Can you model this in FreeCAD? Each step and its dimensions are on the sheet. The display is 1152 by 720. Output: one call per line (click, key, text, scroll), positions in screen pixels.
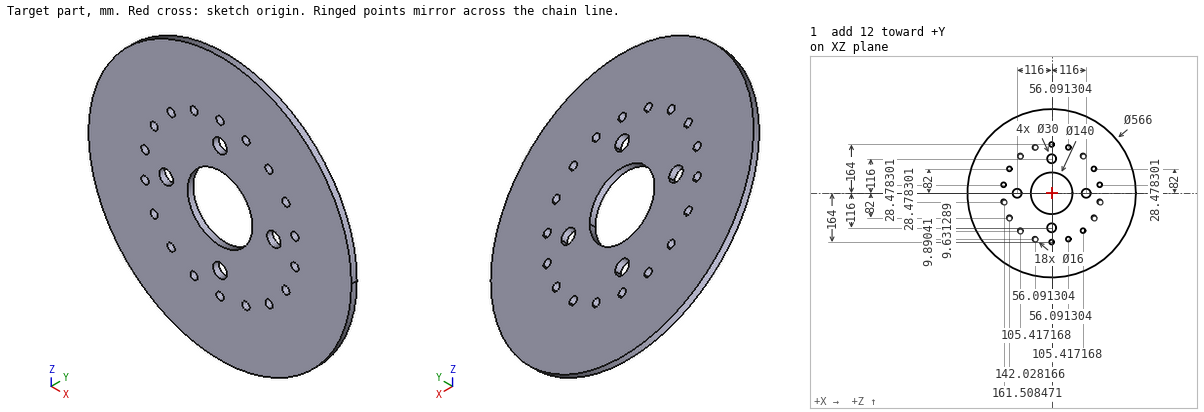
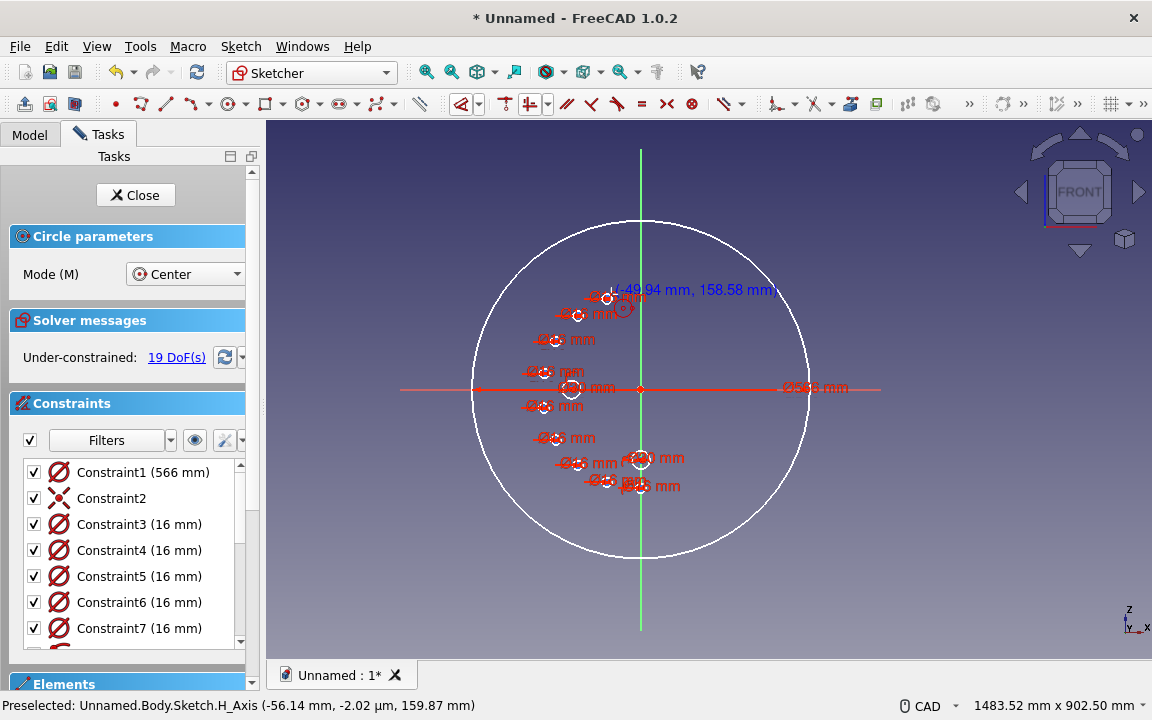
scroll(674, 482, up, 8)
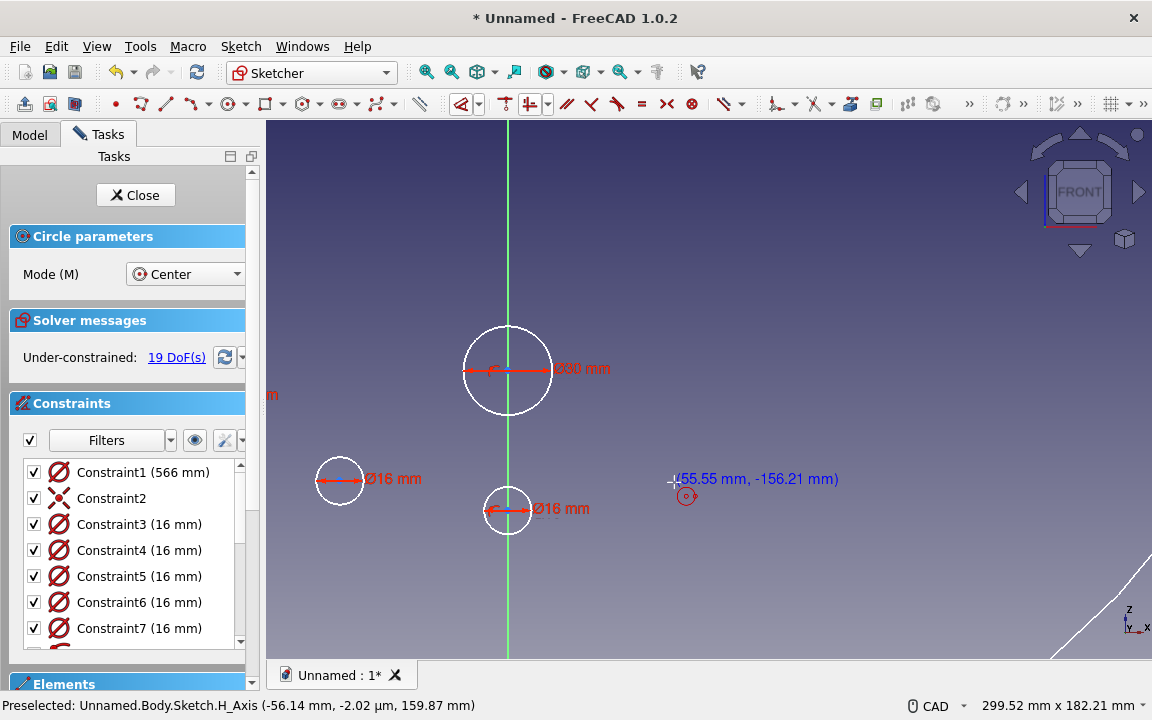
scroll(674, 482, down, 8)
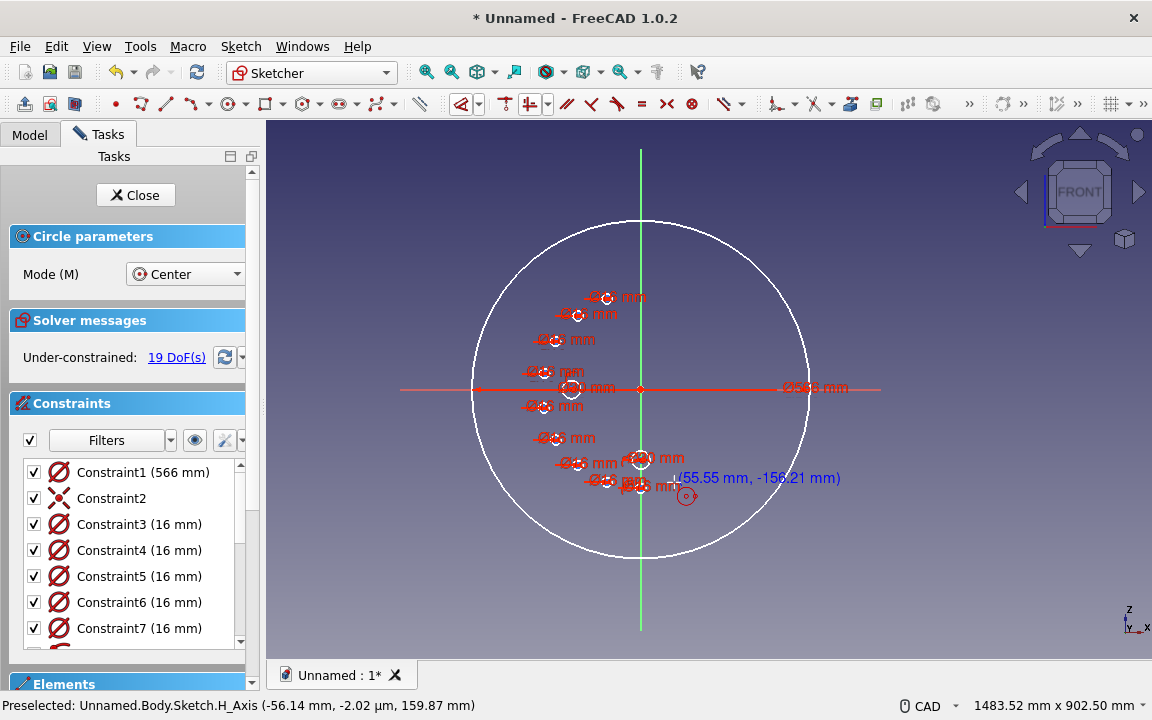
click(674, 482)
move(678, 478)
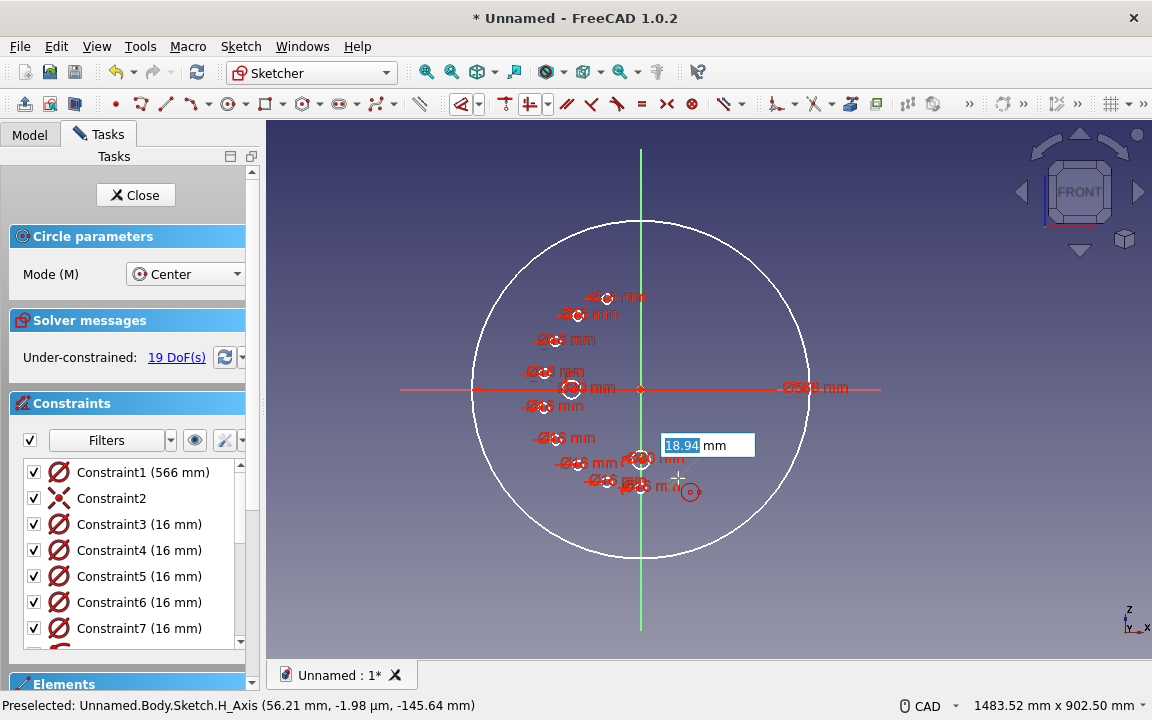
text(16)
key(Return)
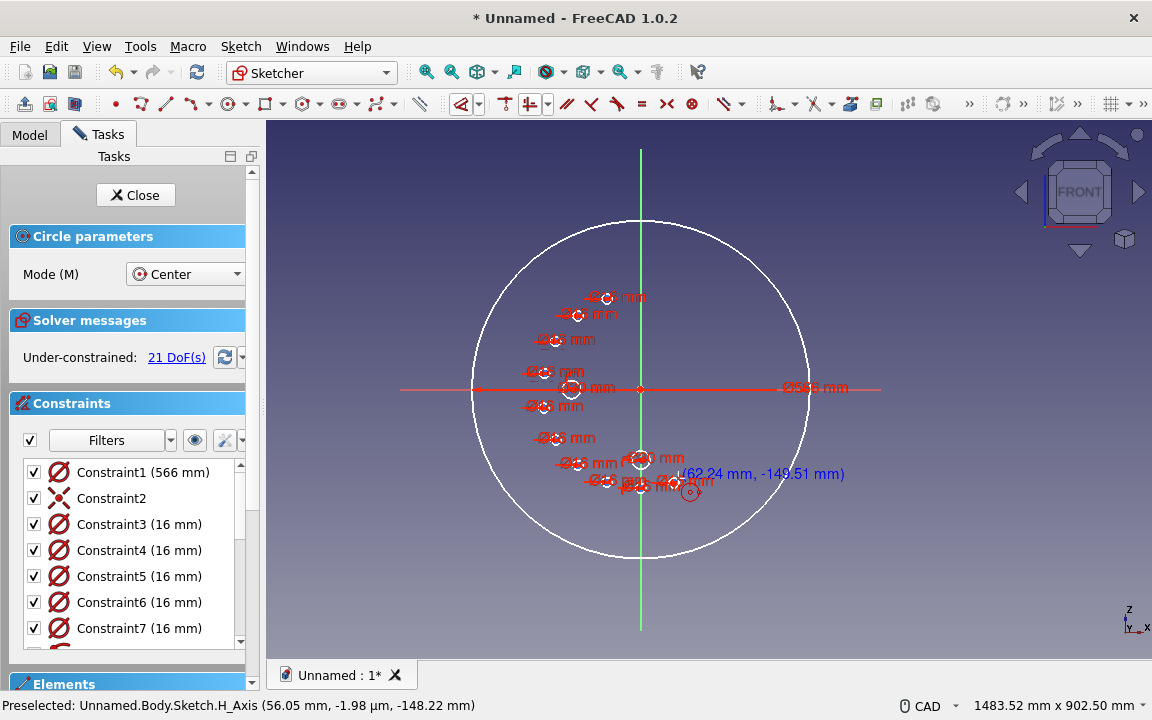
scroll(704, 465, up, 8)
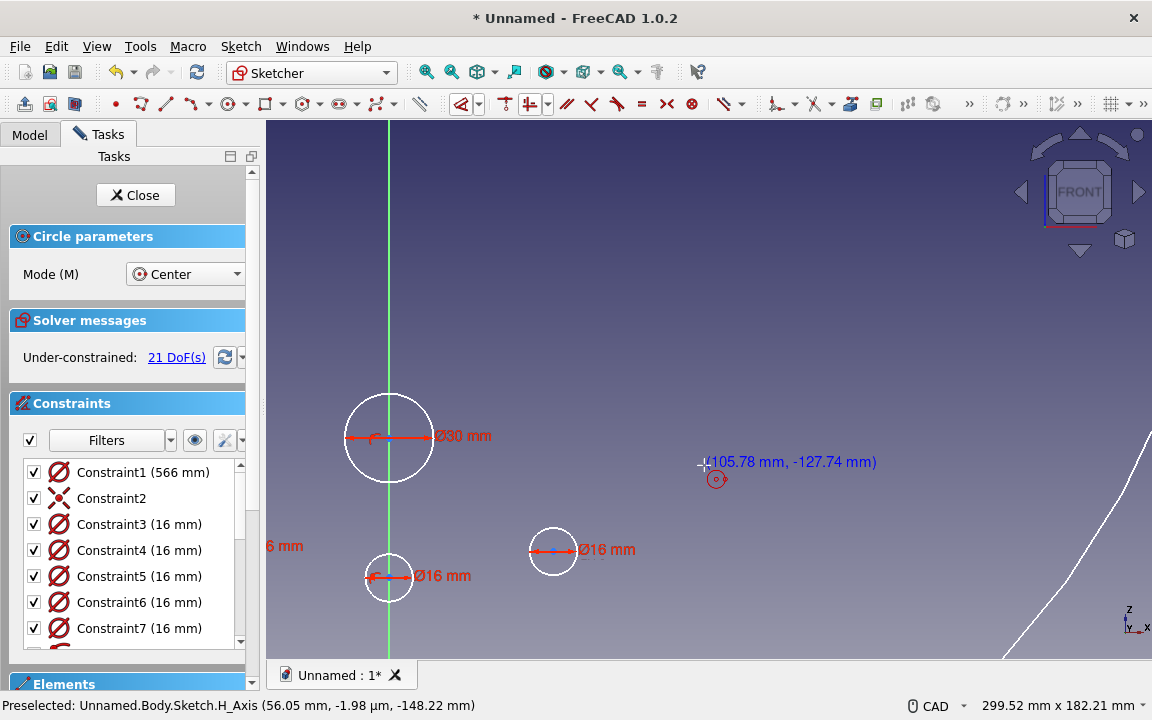
scroll(704, 465, down, 8)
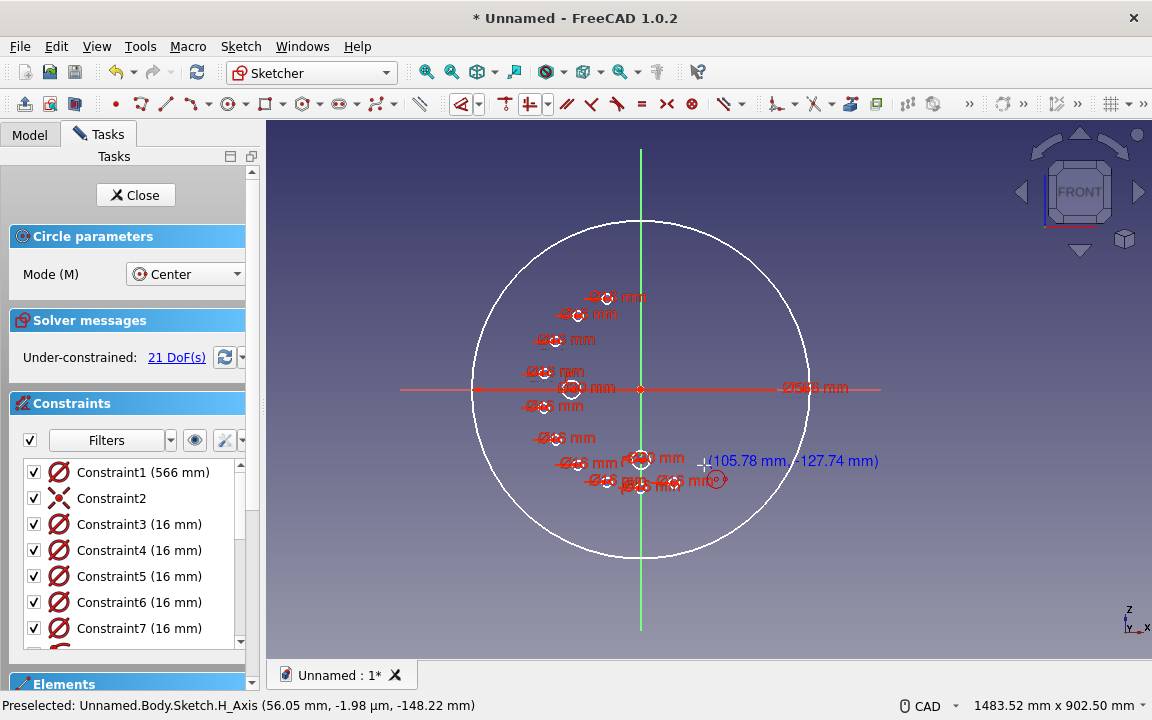
click(704, 465)
move(707, 461)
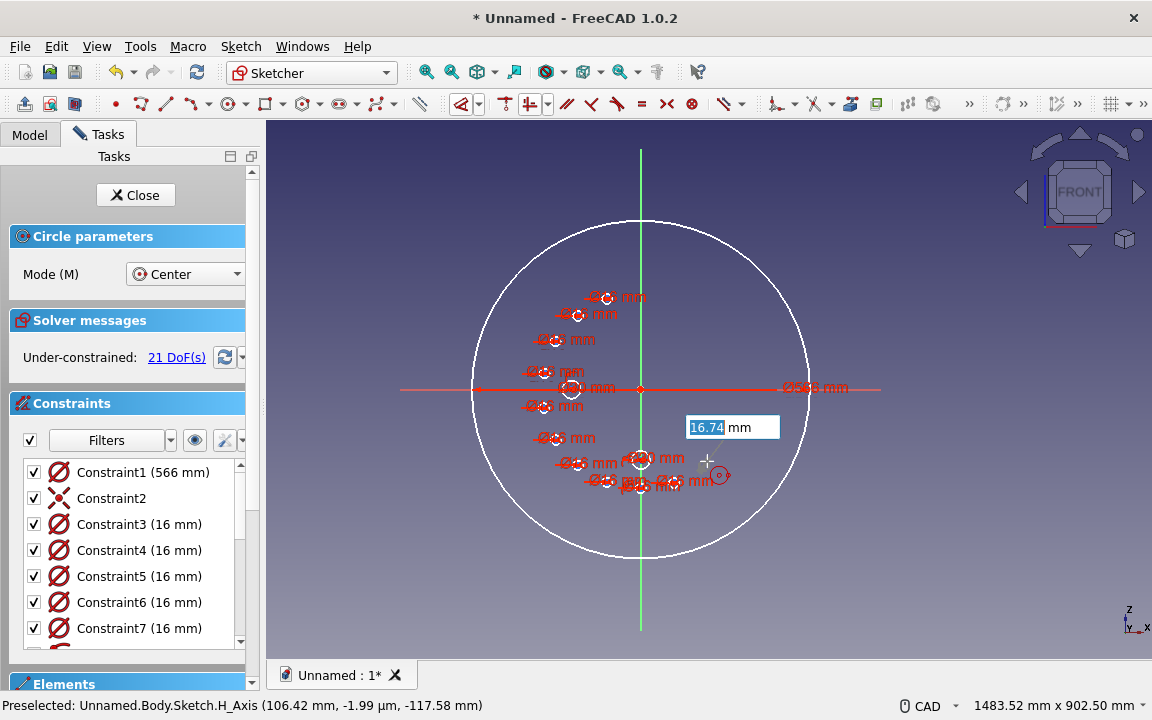
text(16)
key(Return)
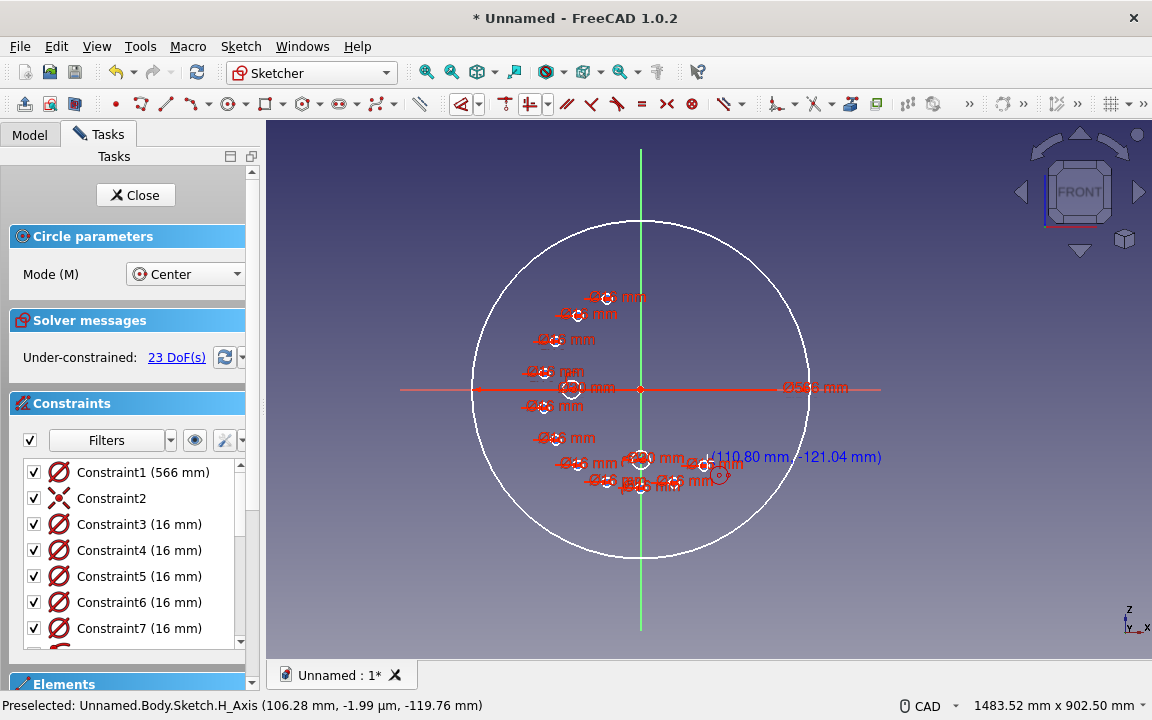
scroll(710, 390, up, 5)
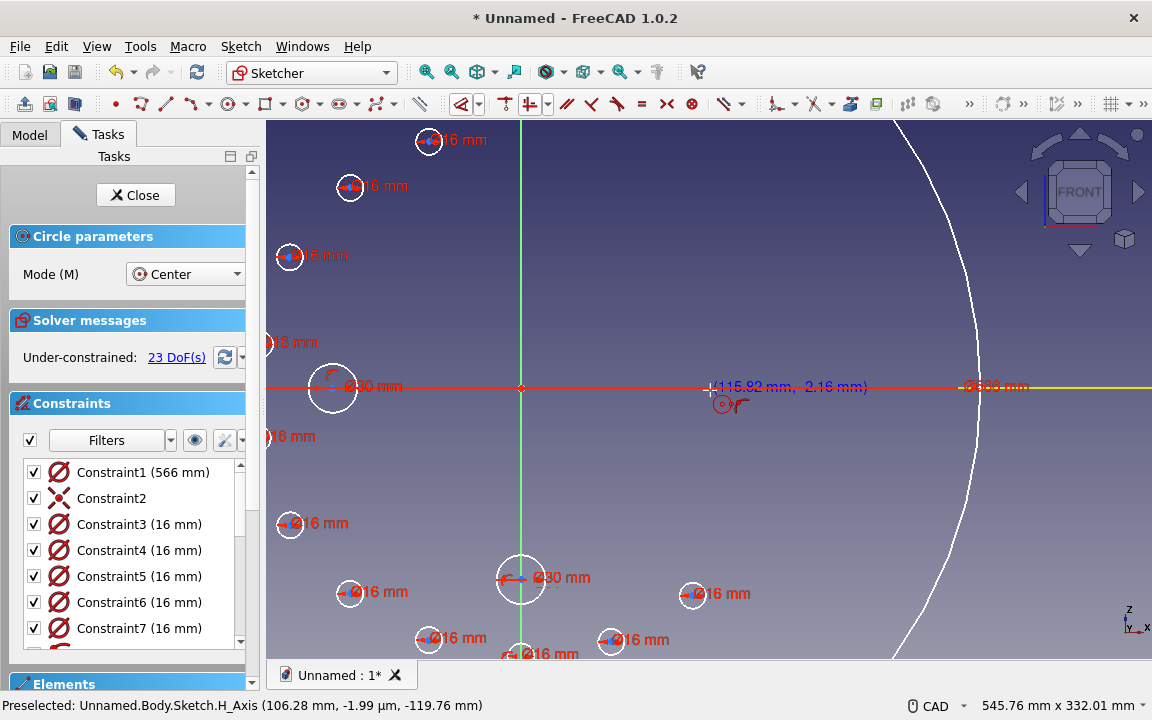
click(709, 388)
move(727, 371)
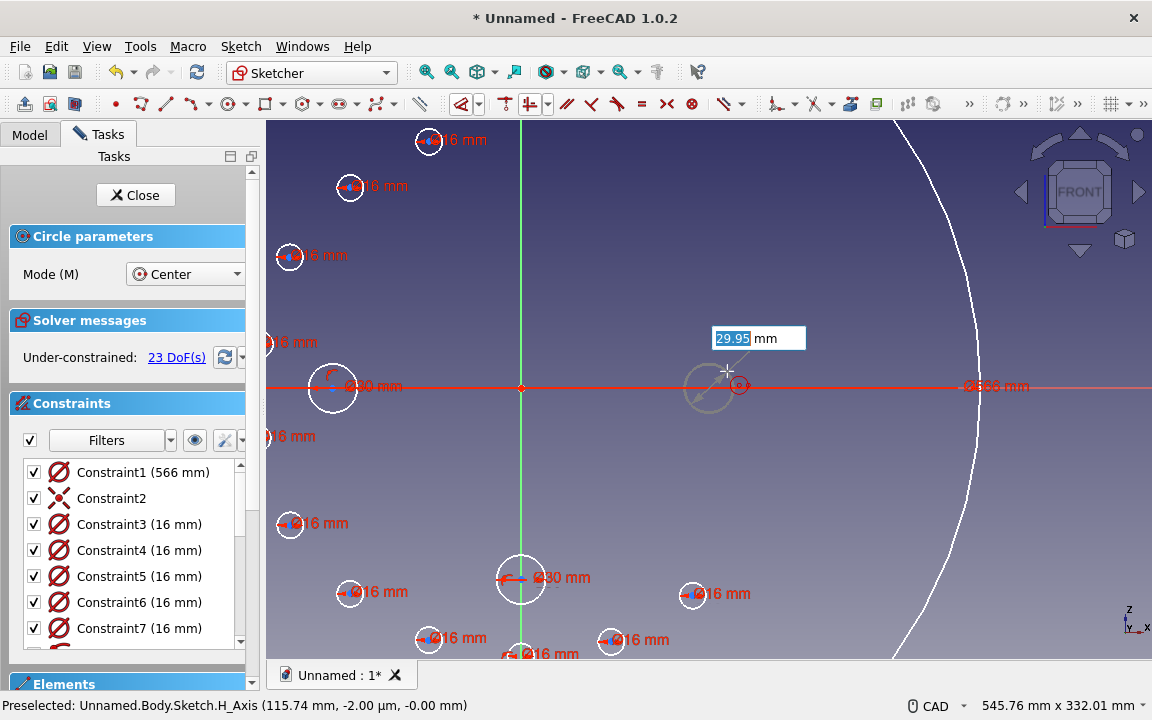
text(30)
key(Return)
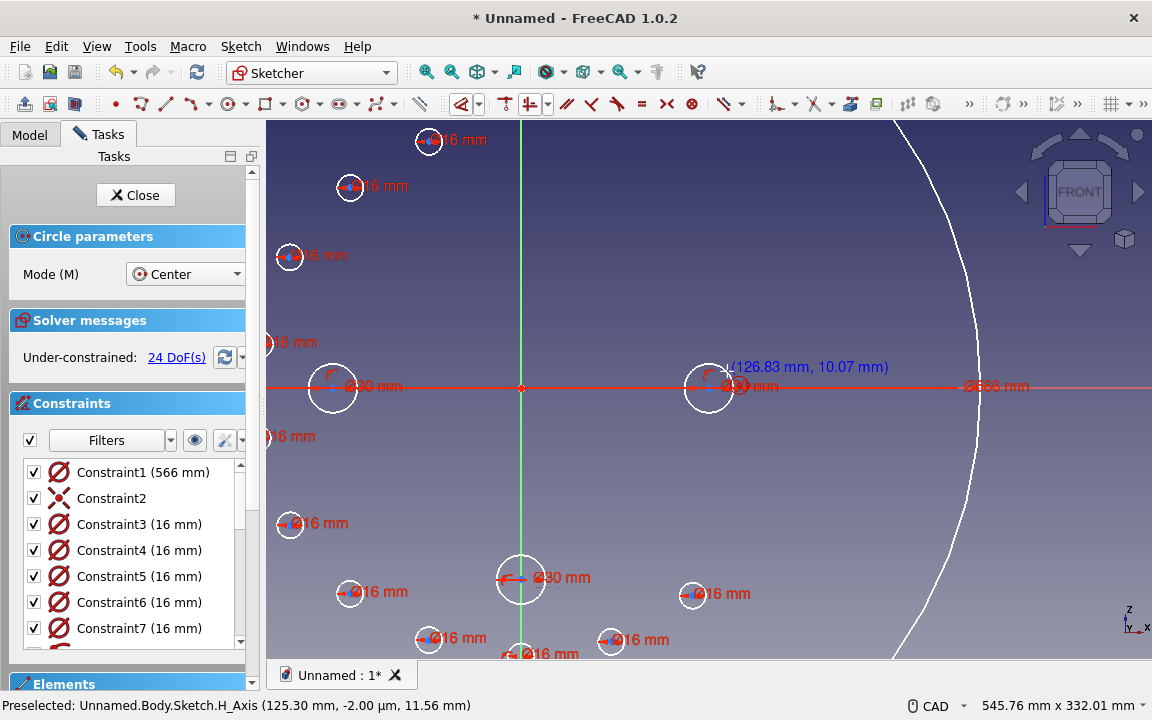
scroll(752, 521, up, 3)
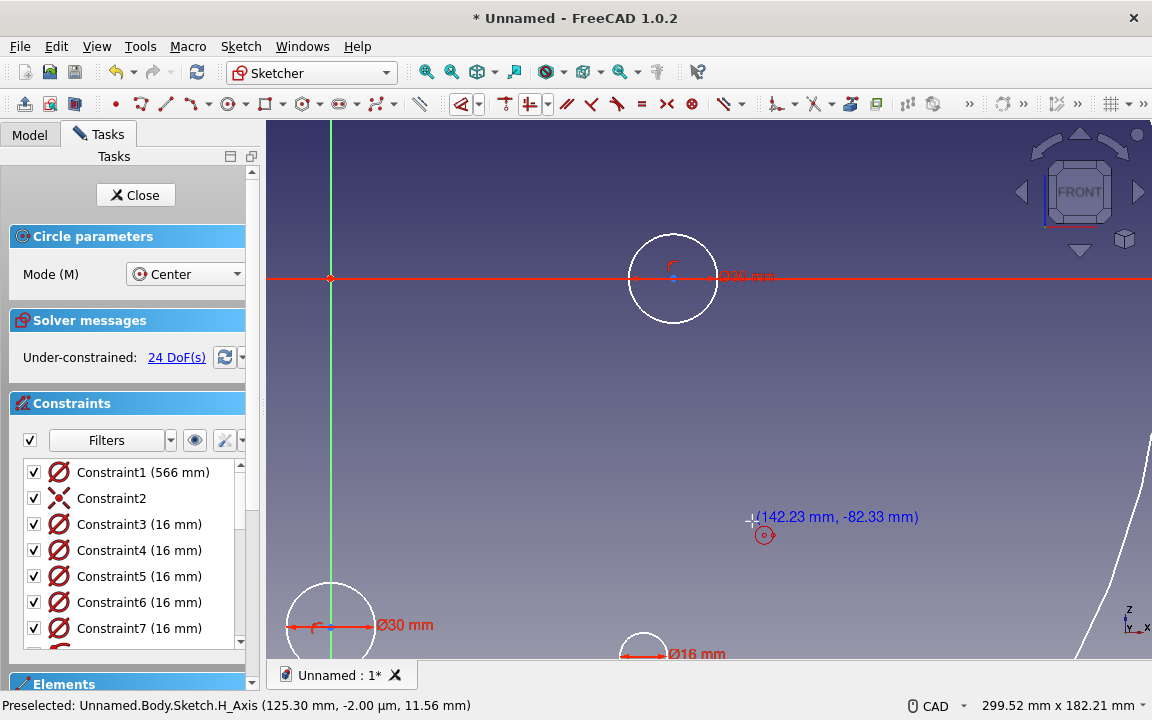
scroll(719, 418, down, 8)